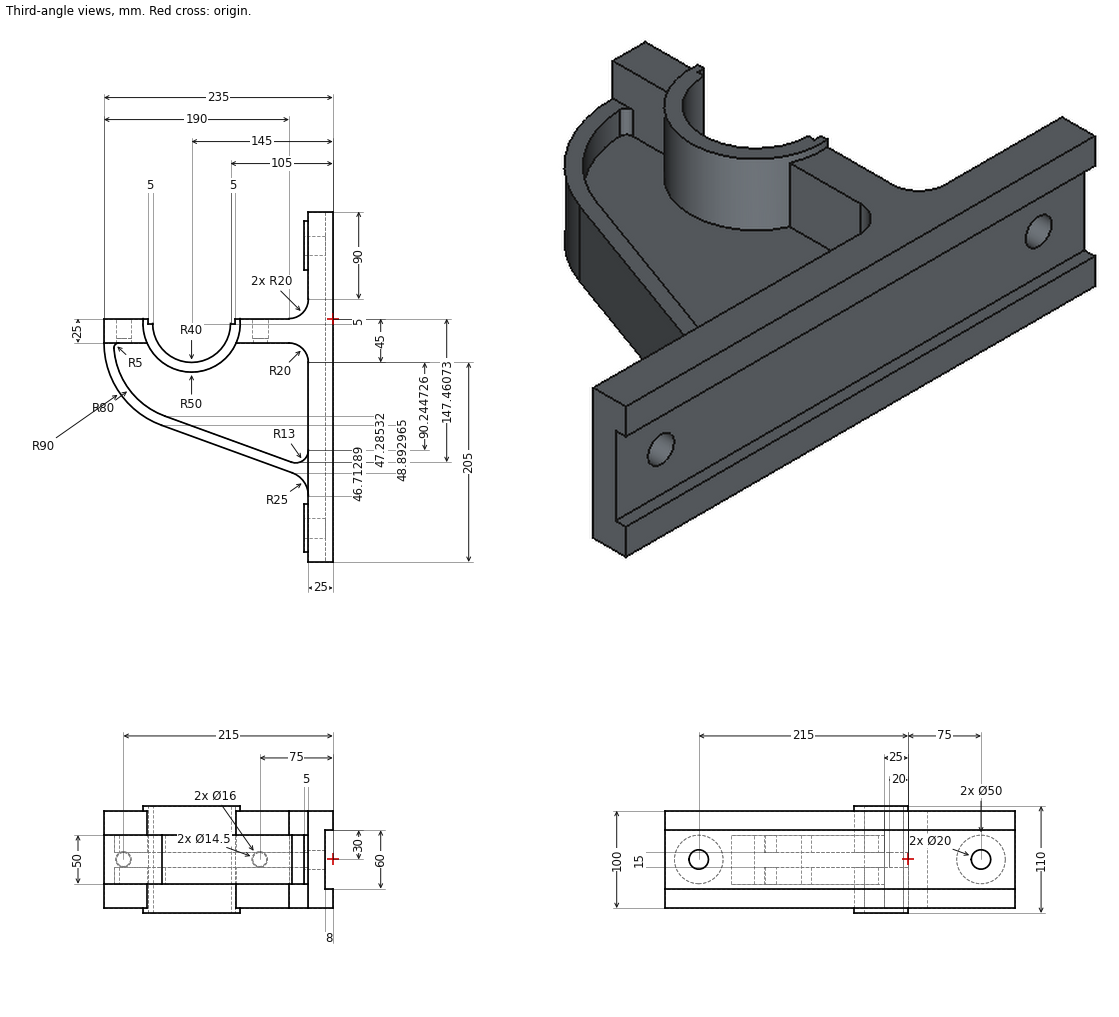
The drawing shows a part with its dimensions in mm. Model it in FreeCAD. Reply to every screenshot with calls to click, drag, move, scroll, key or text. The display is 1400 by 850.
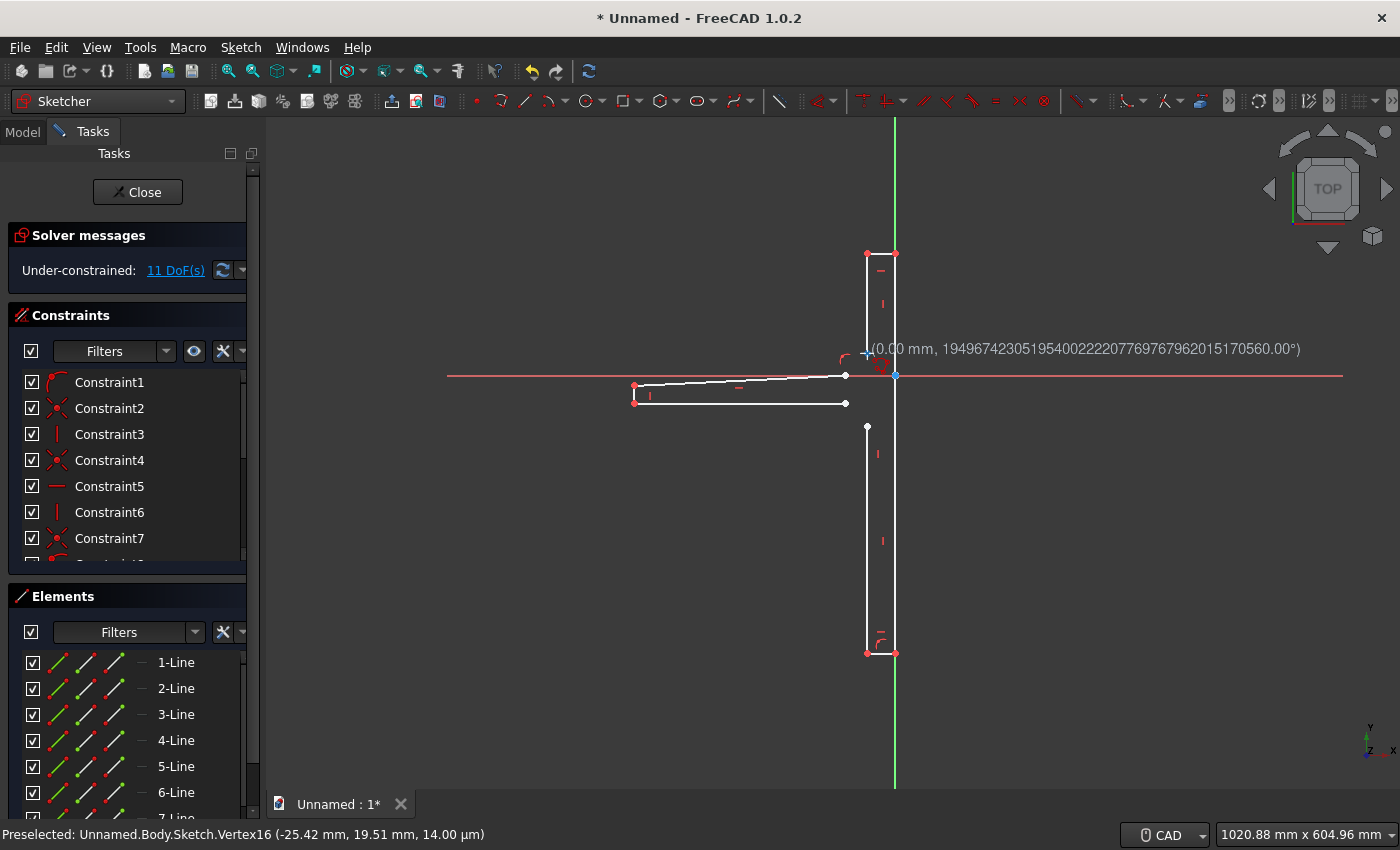
key(g)
key(3)
key(a)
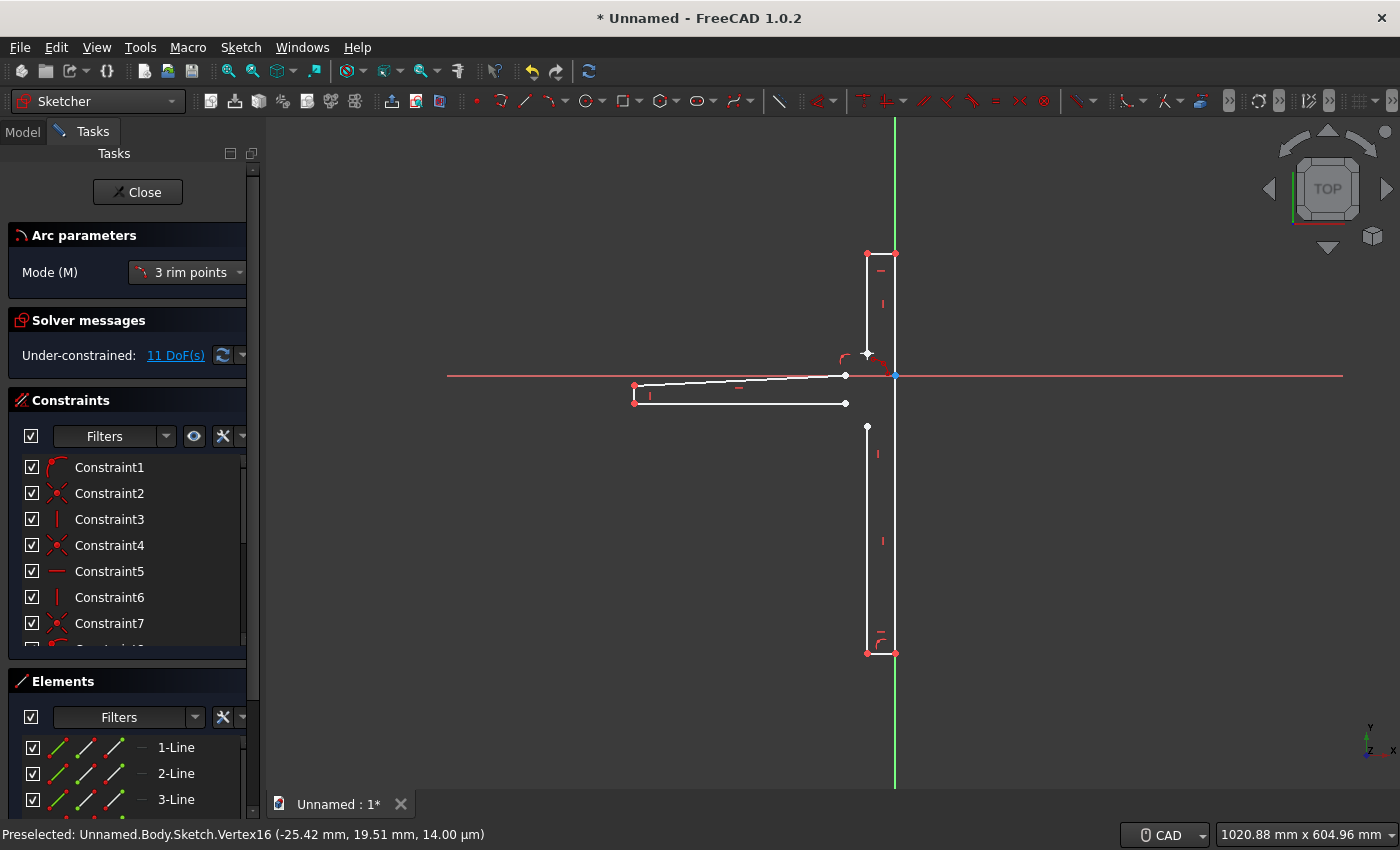
click(845, 404)
click(867, 427)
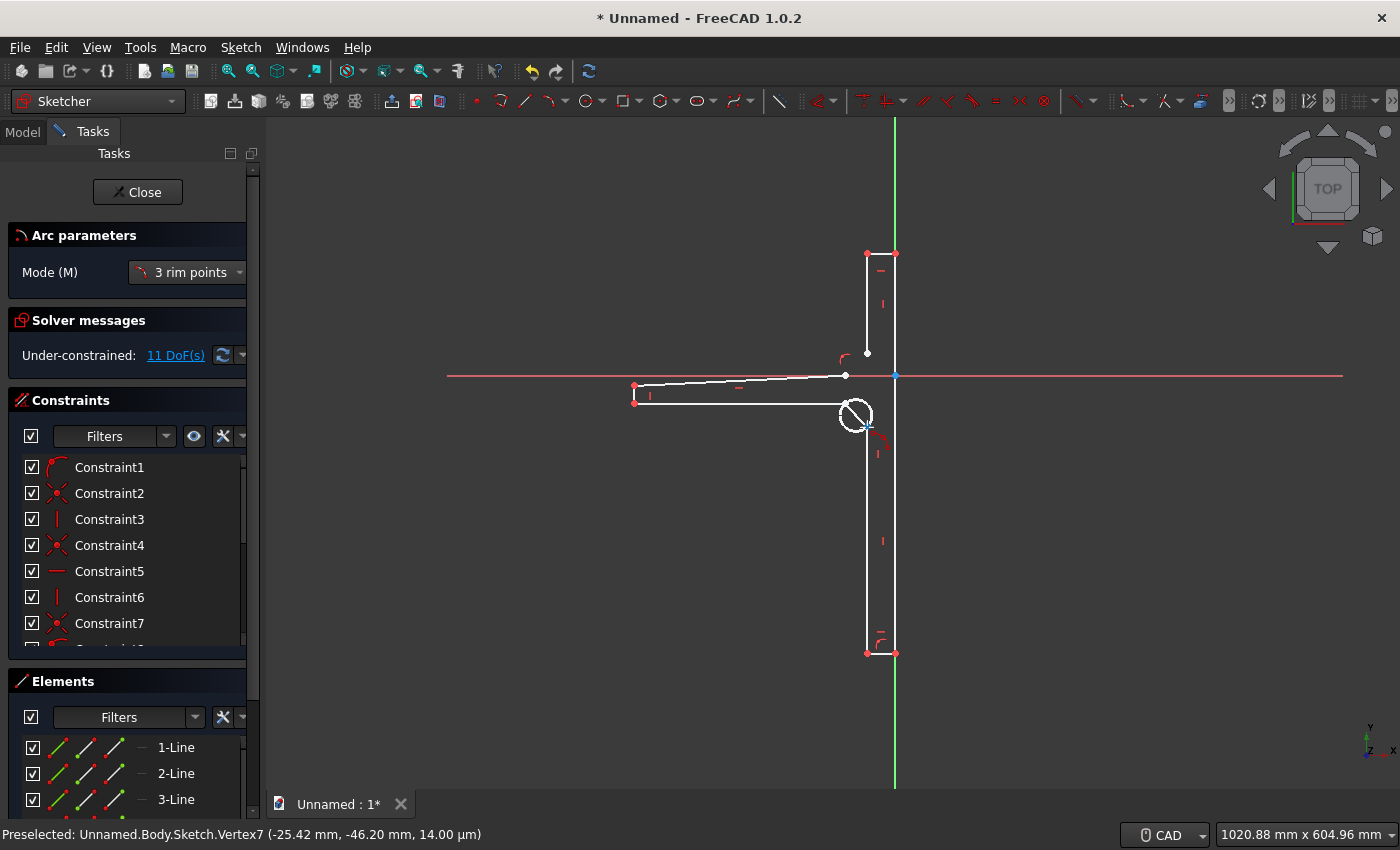
scroll(861, 410, up, 5)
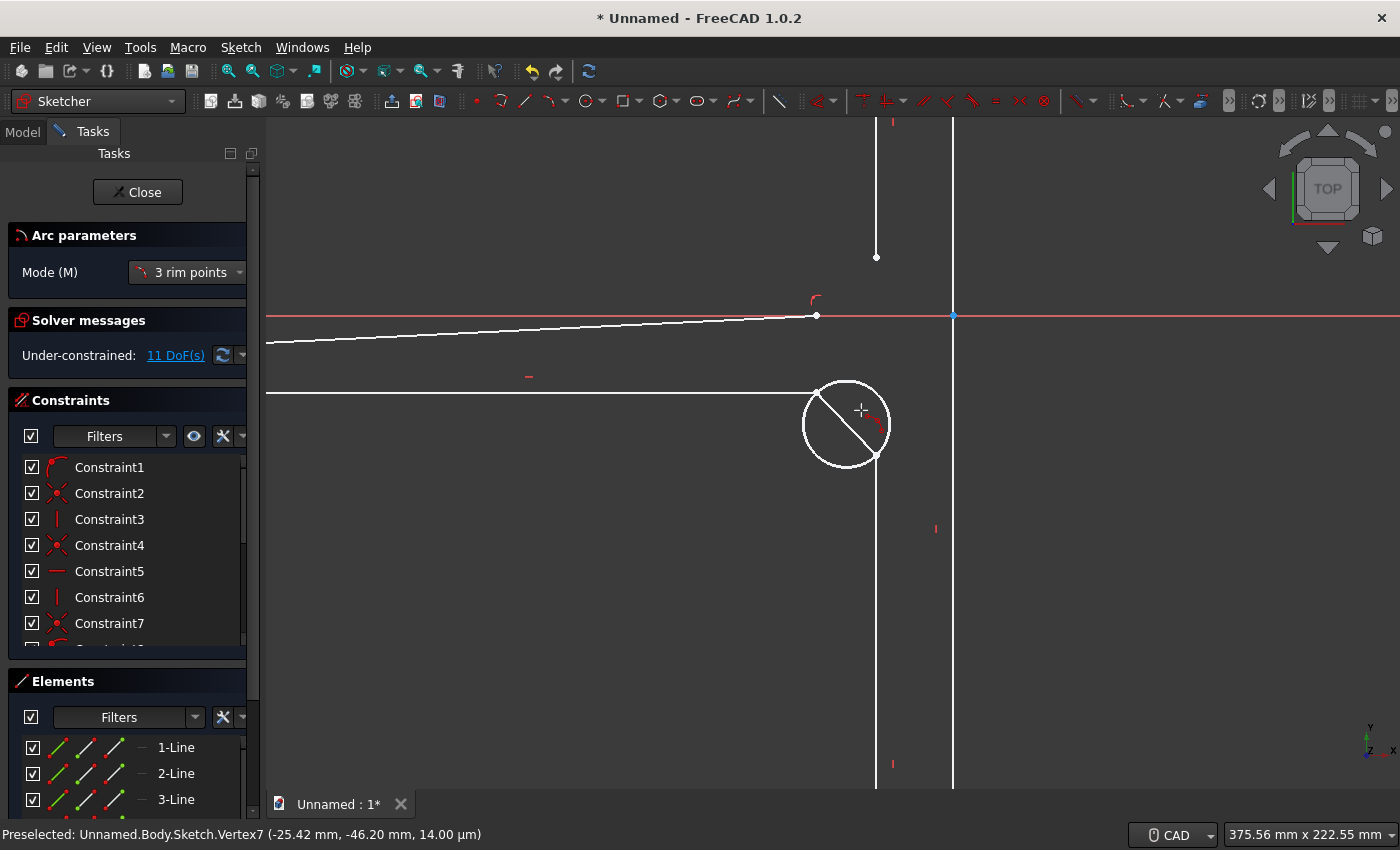
click(860, 409)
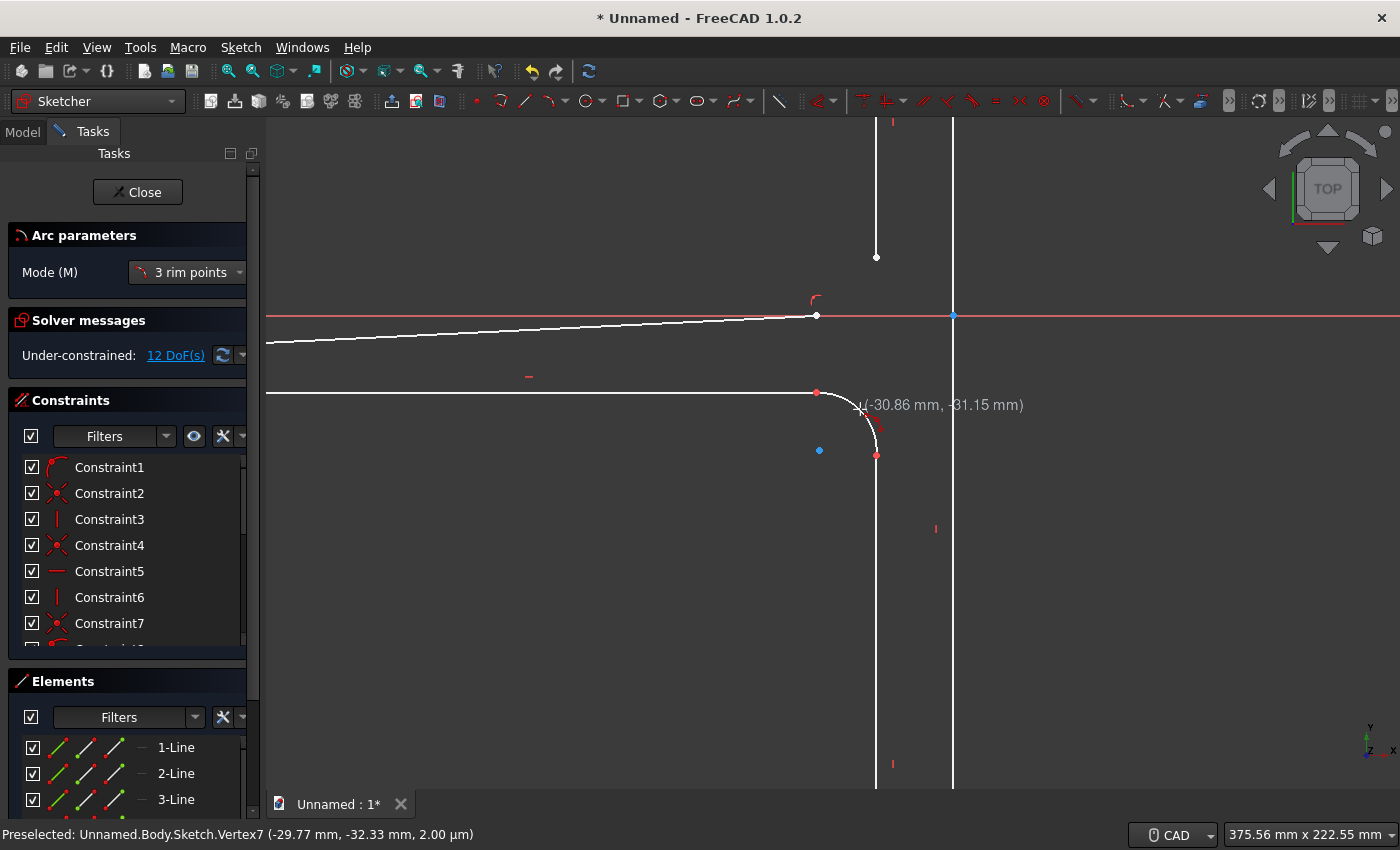
click(876, 257)
click(817, 316)
click(860, 298)
key(Escape)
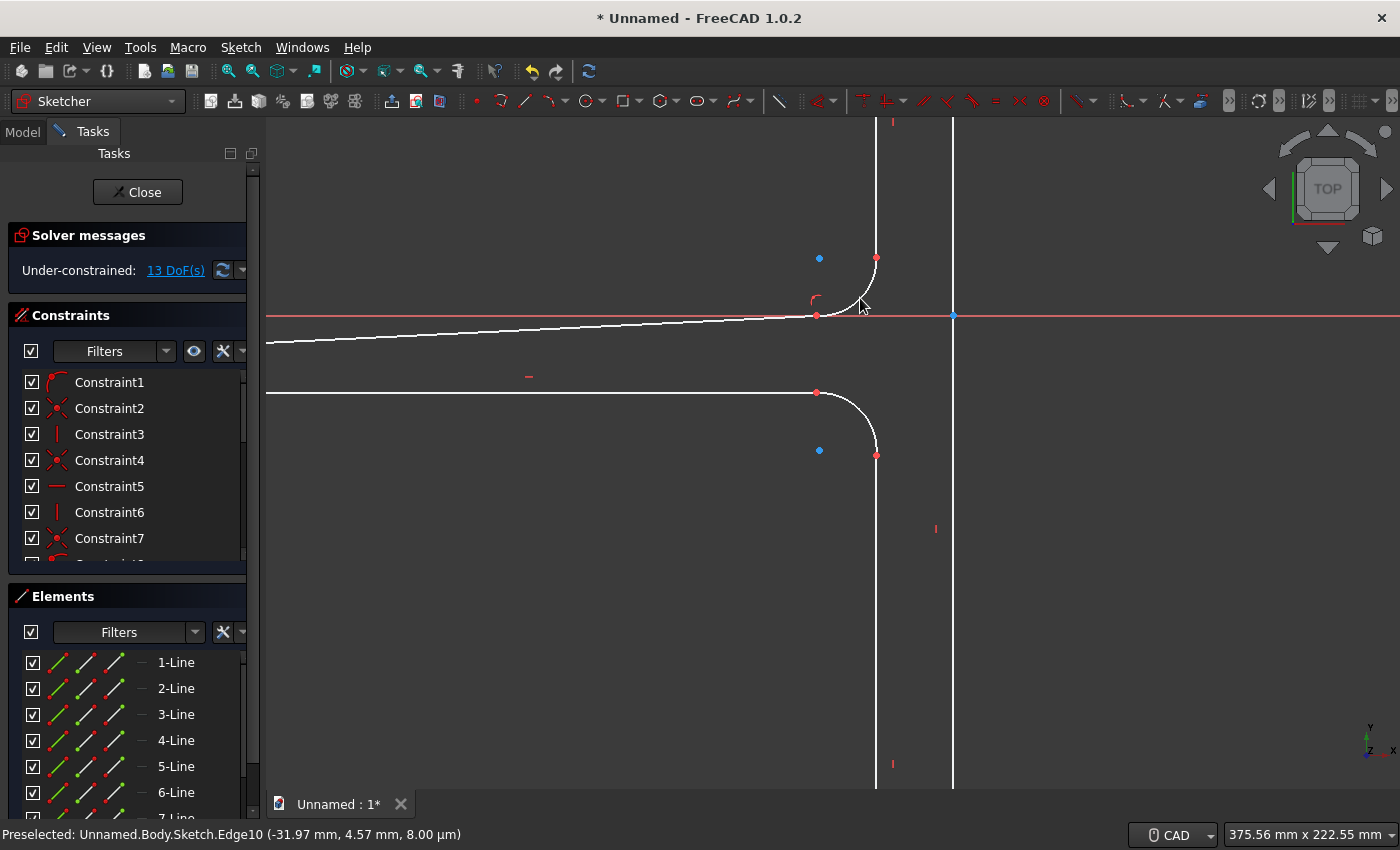
click(415, 336)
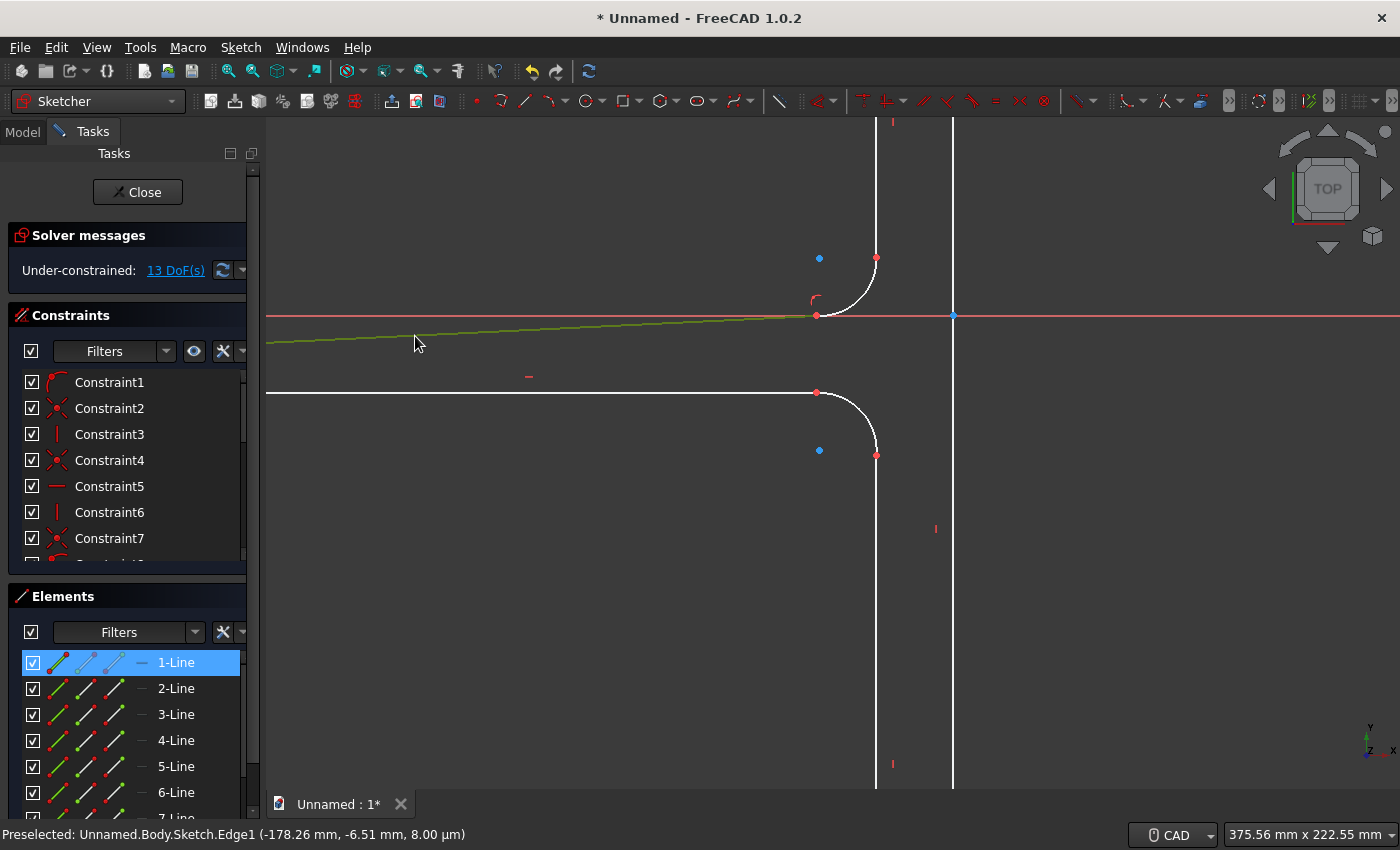
click(870, 284)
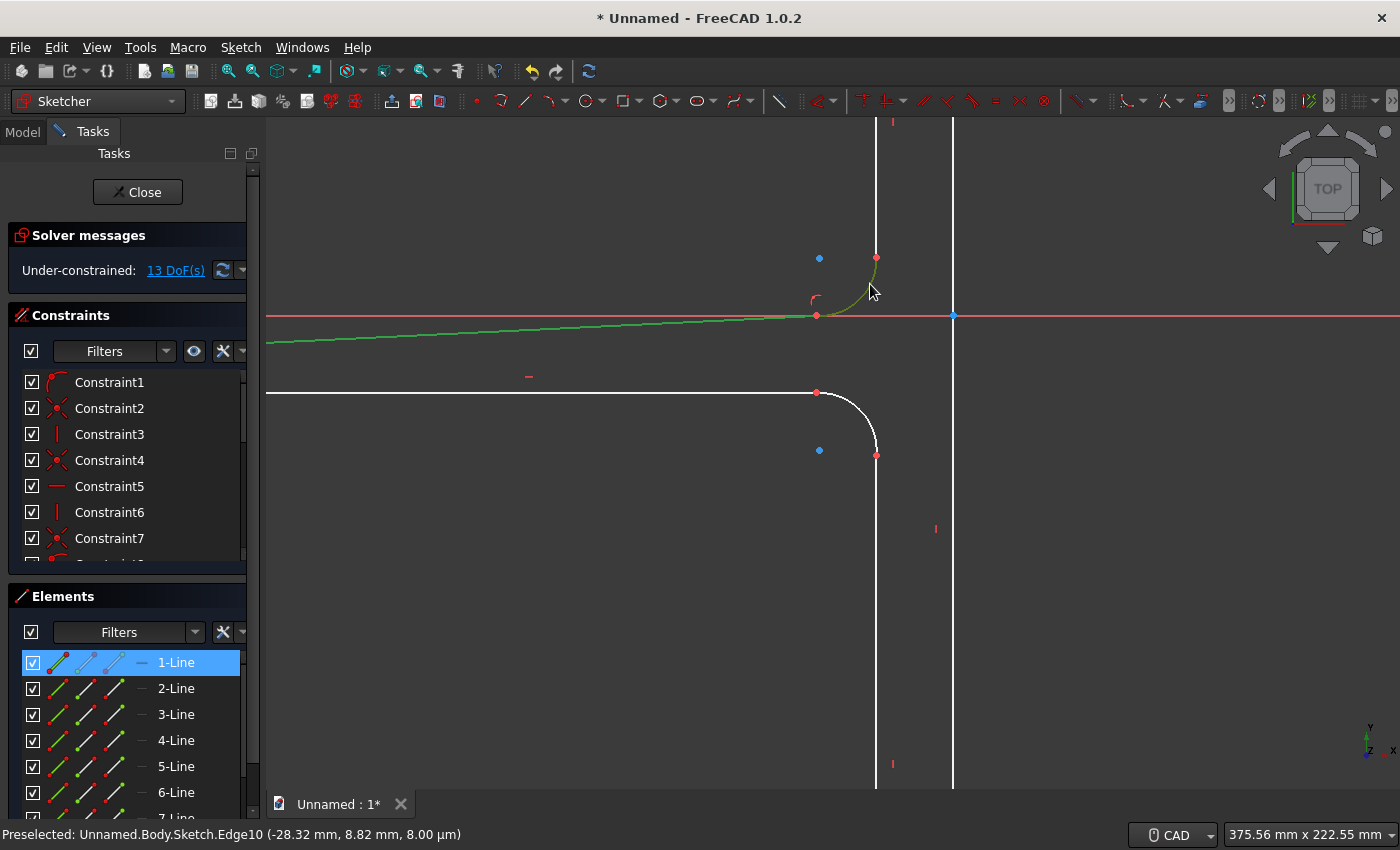
click(972, 102)